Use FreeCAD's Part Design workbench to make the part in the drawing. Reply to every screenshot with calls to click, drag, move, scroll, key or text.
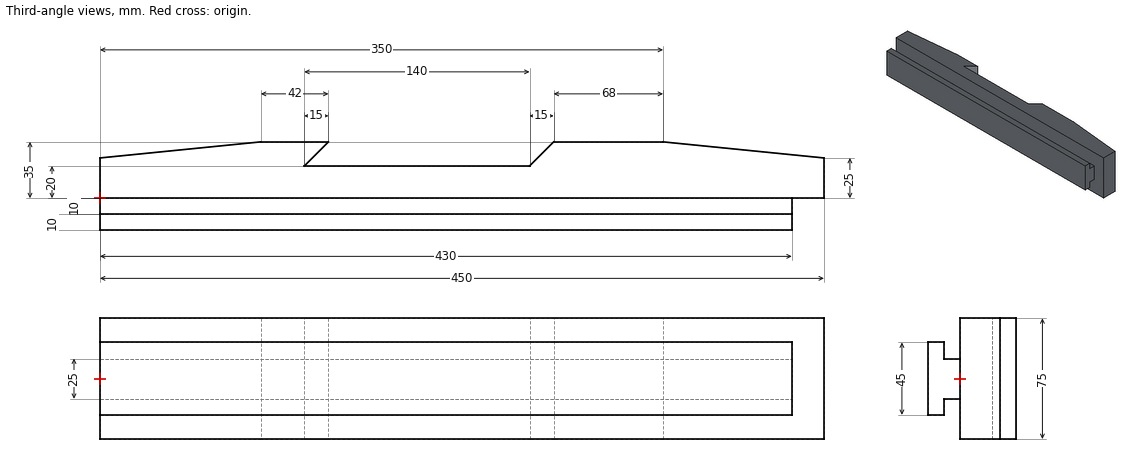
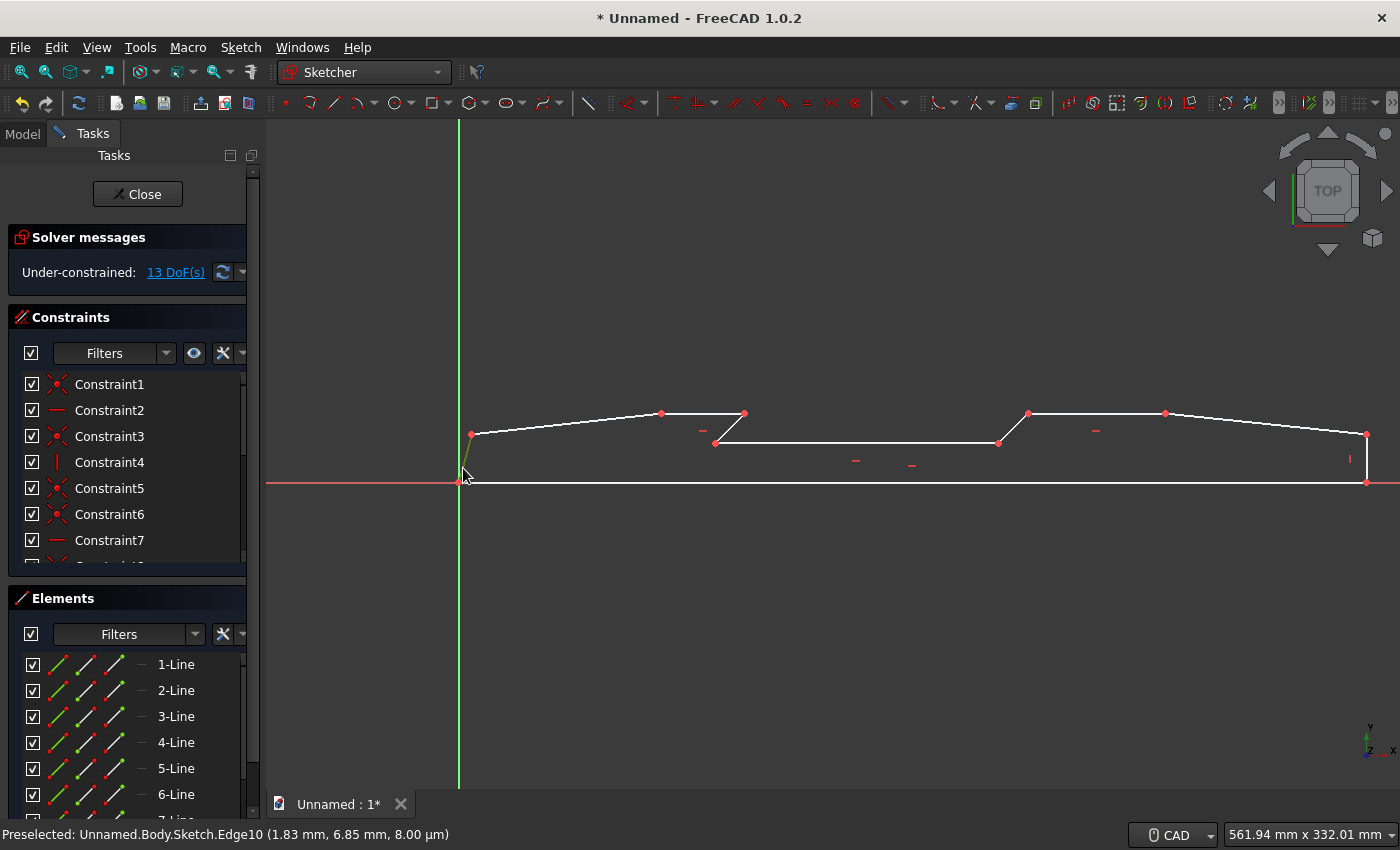
click(716, 104)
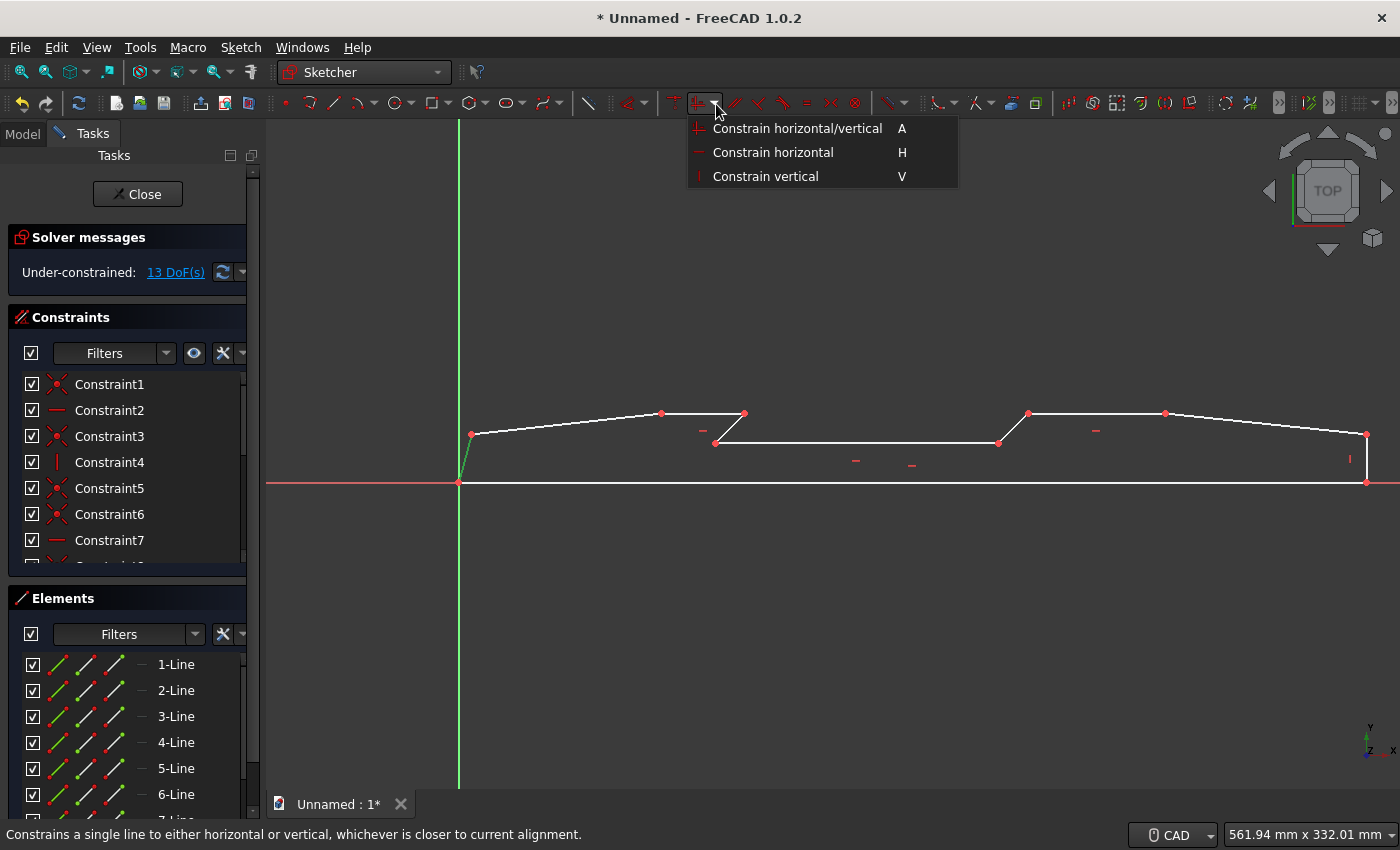
click(823, 176)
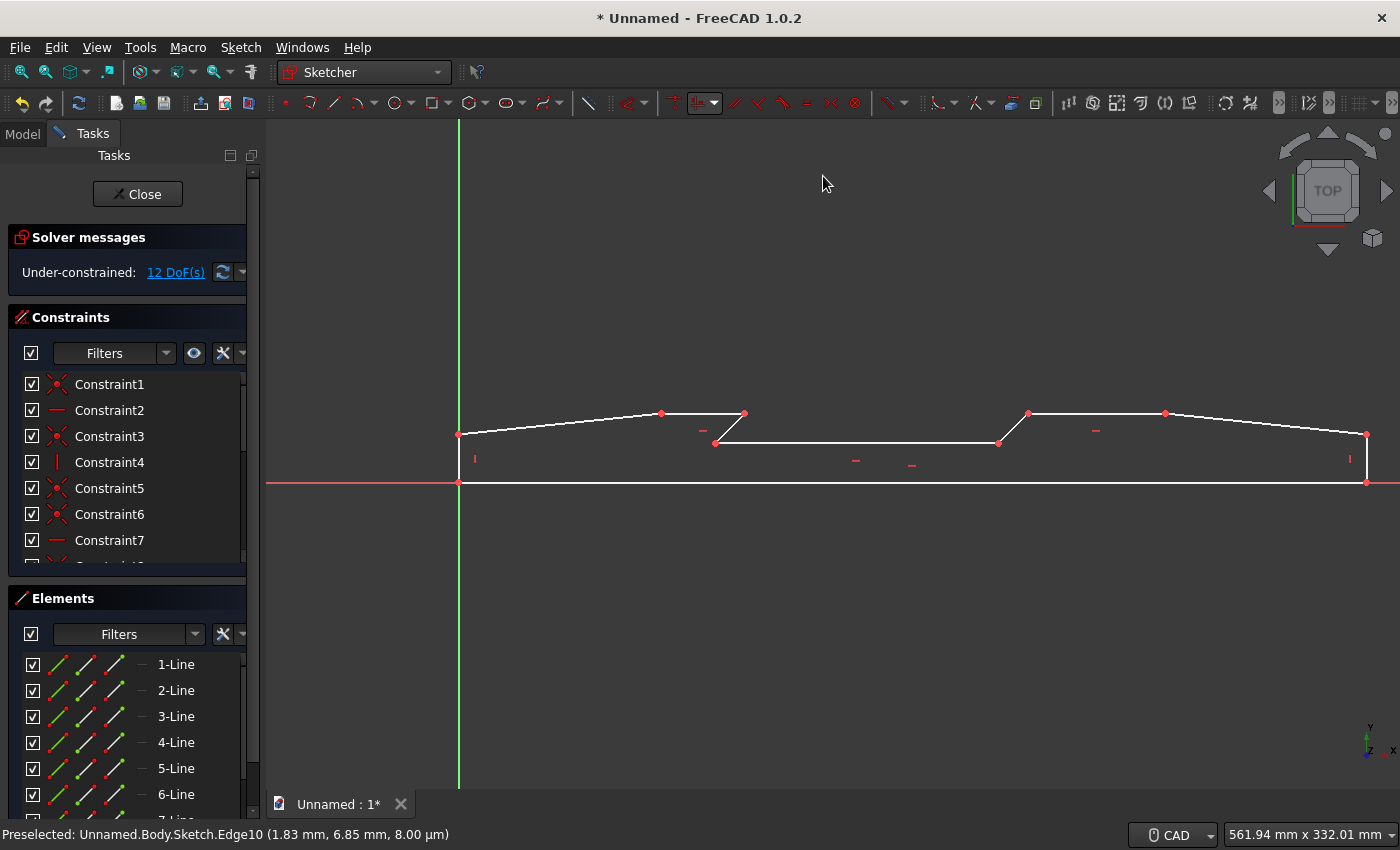
scroll(463, 467, down, 2)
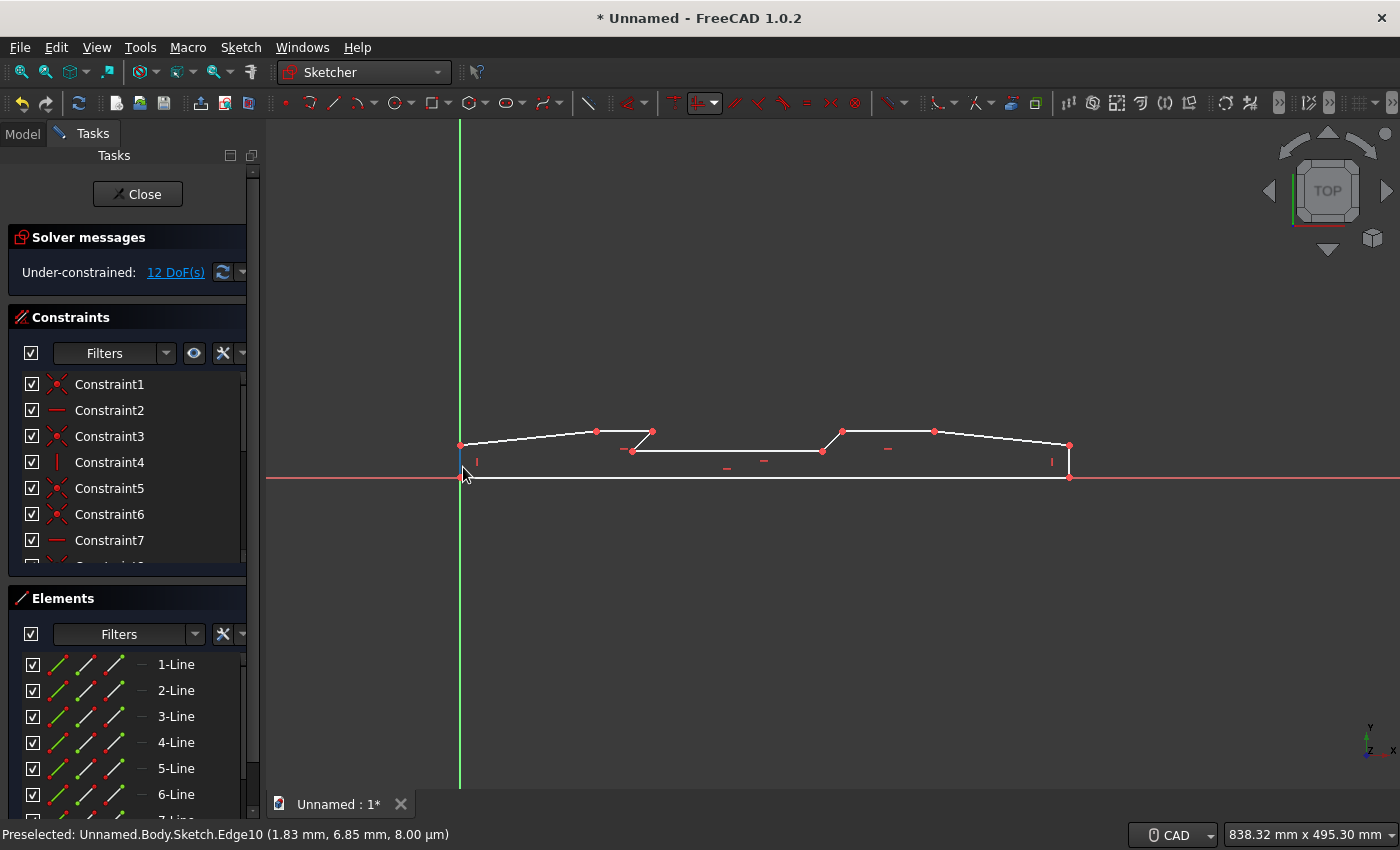
scroll(1069, 468, up, 2)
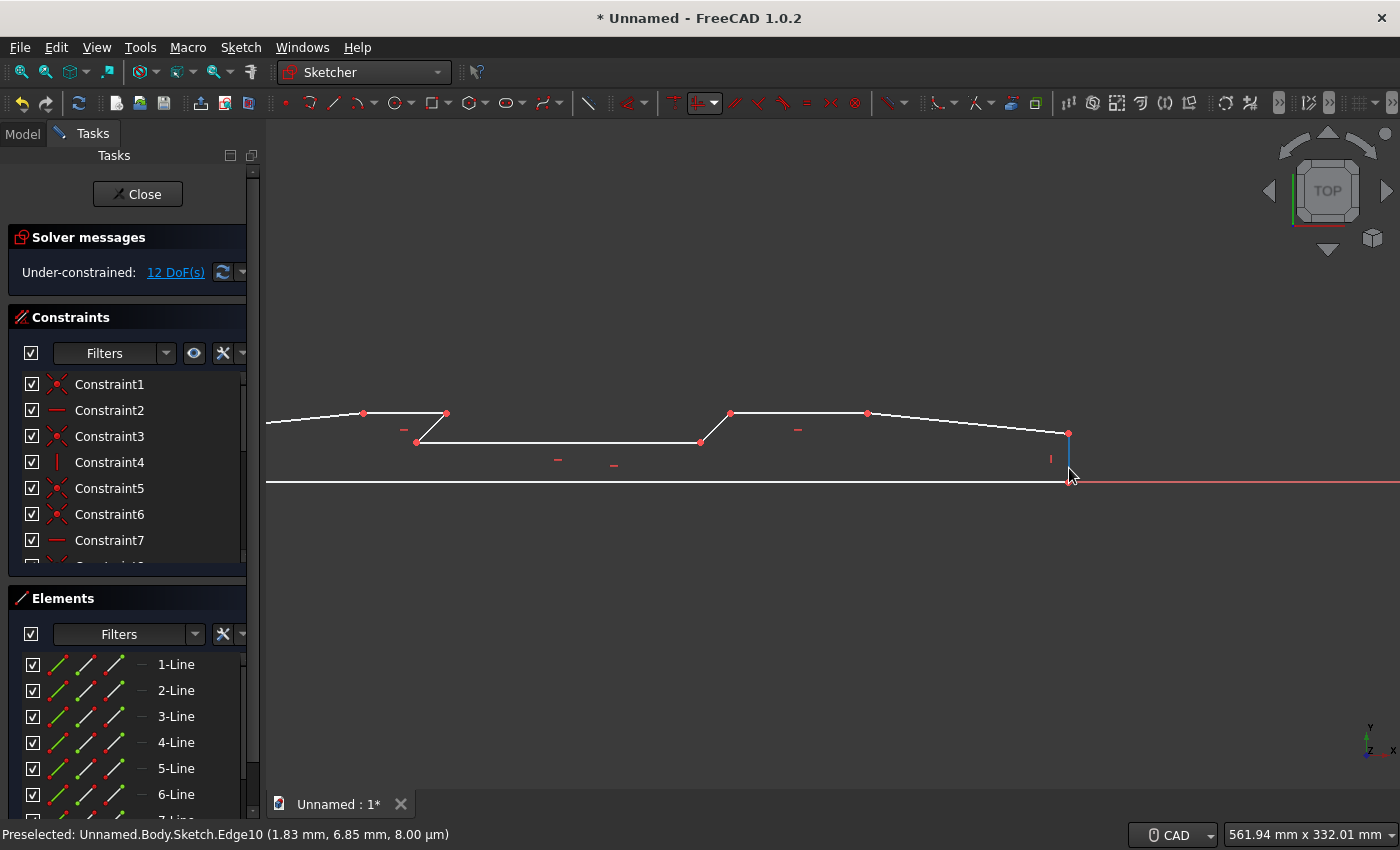
click(1069, 468)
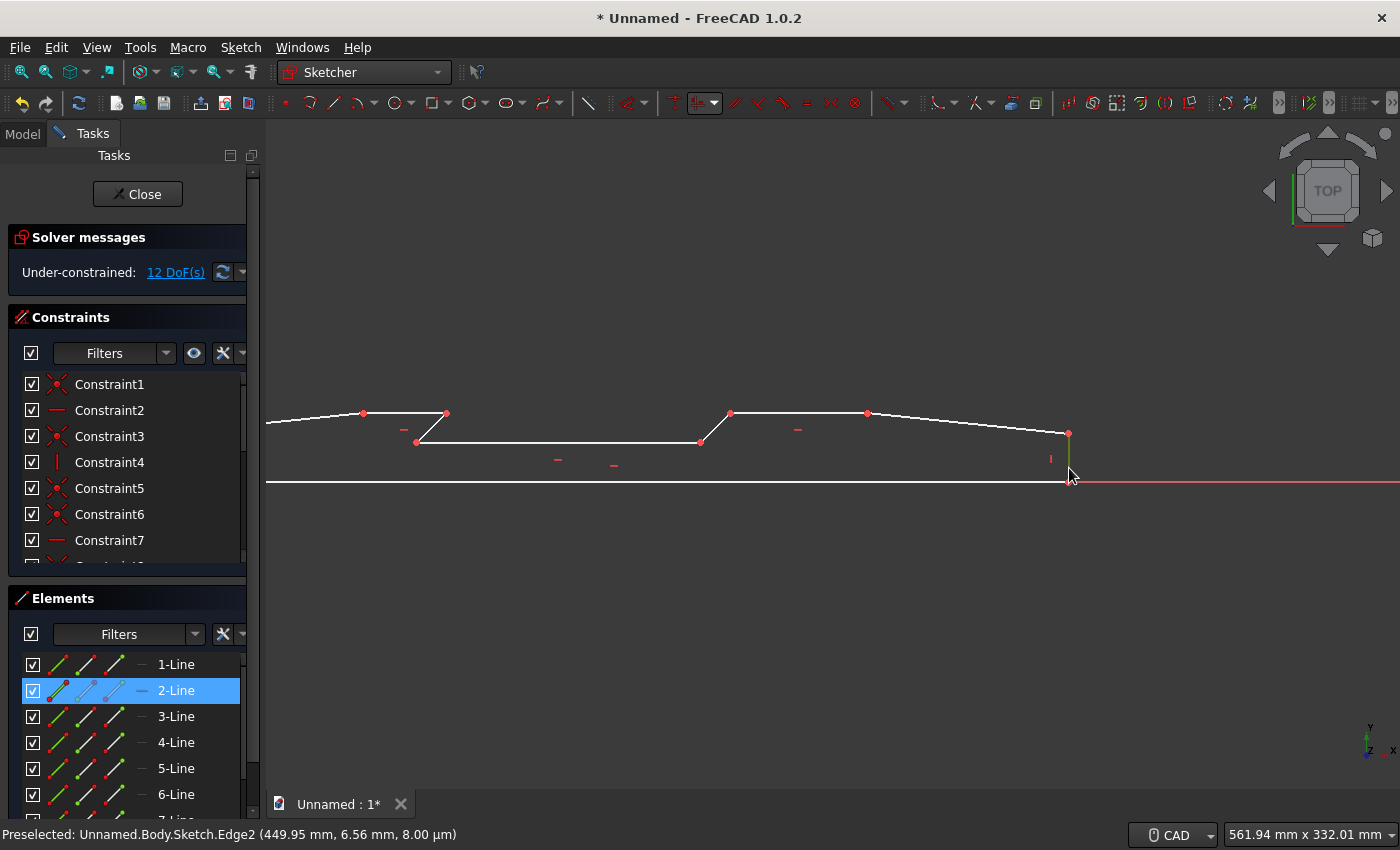
key(i)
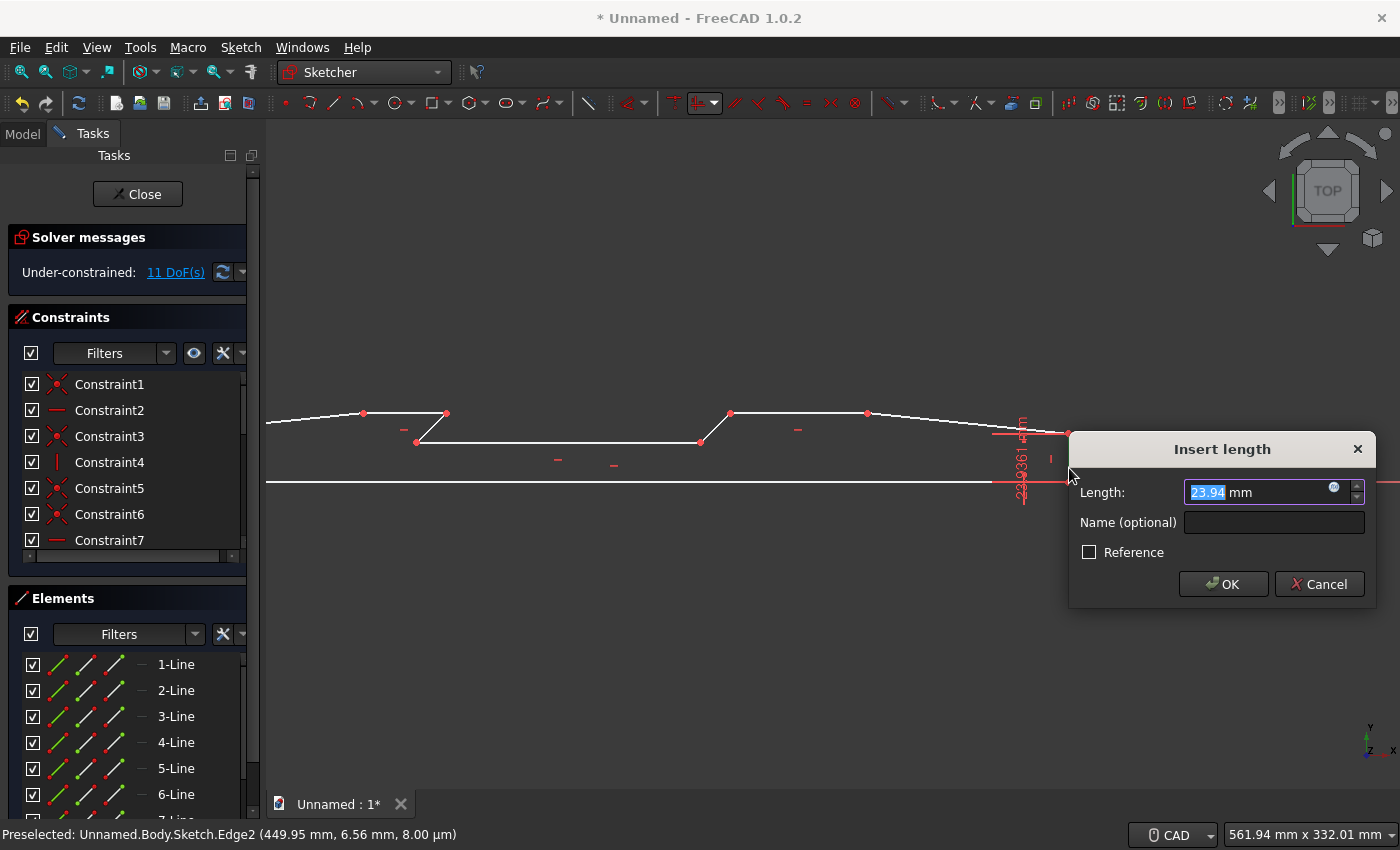
text(25)
key(Return)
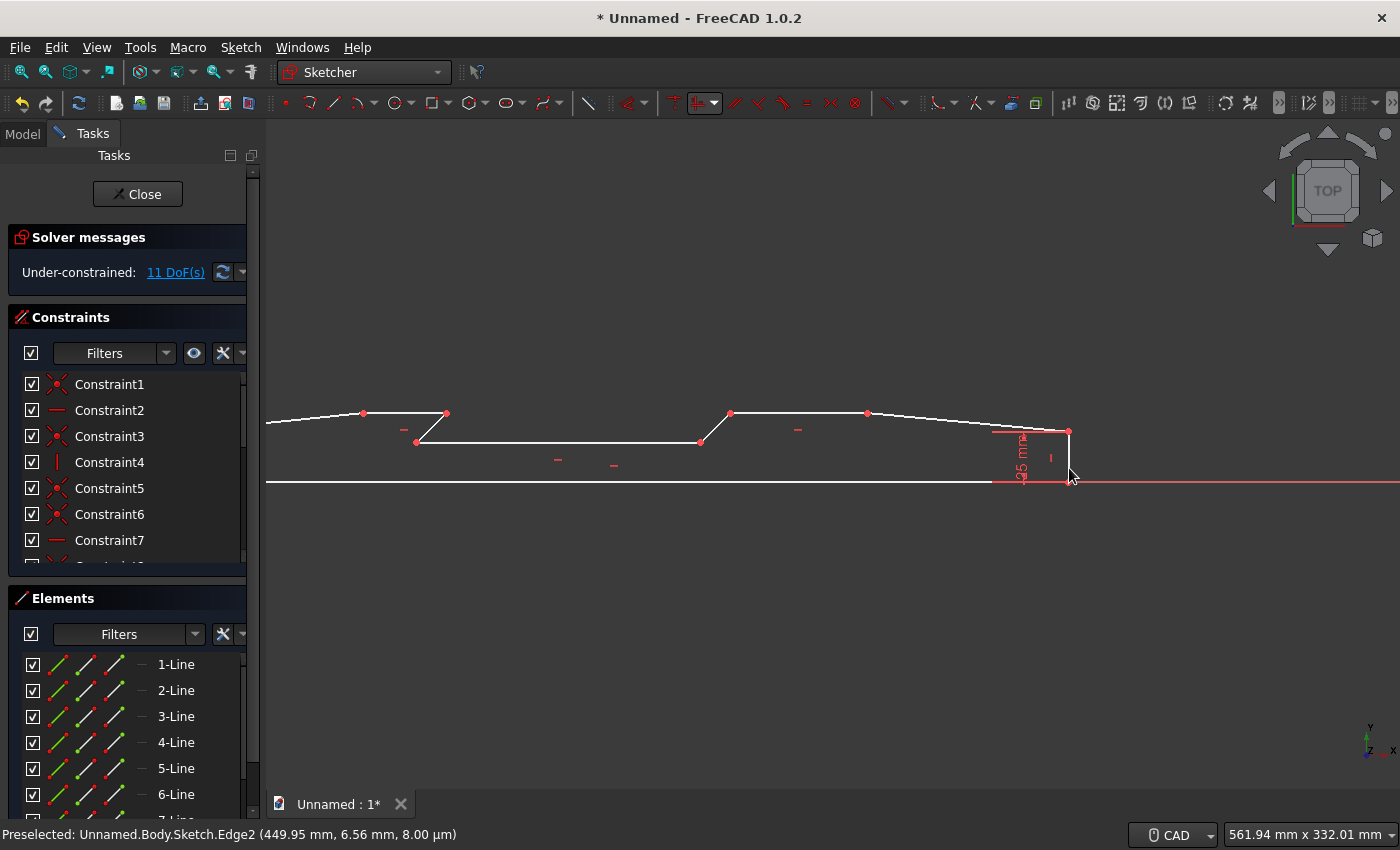
click(826, 413)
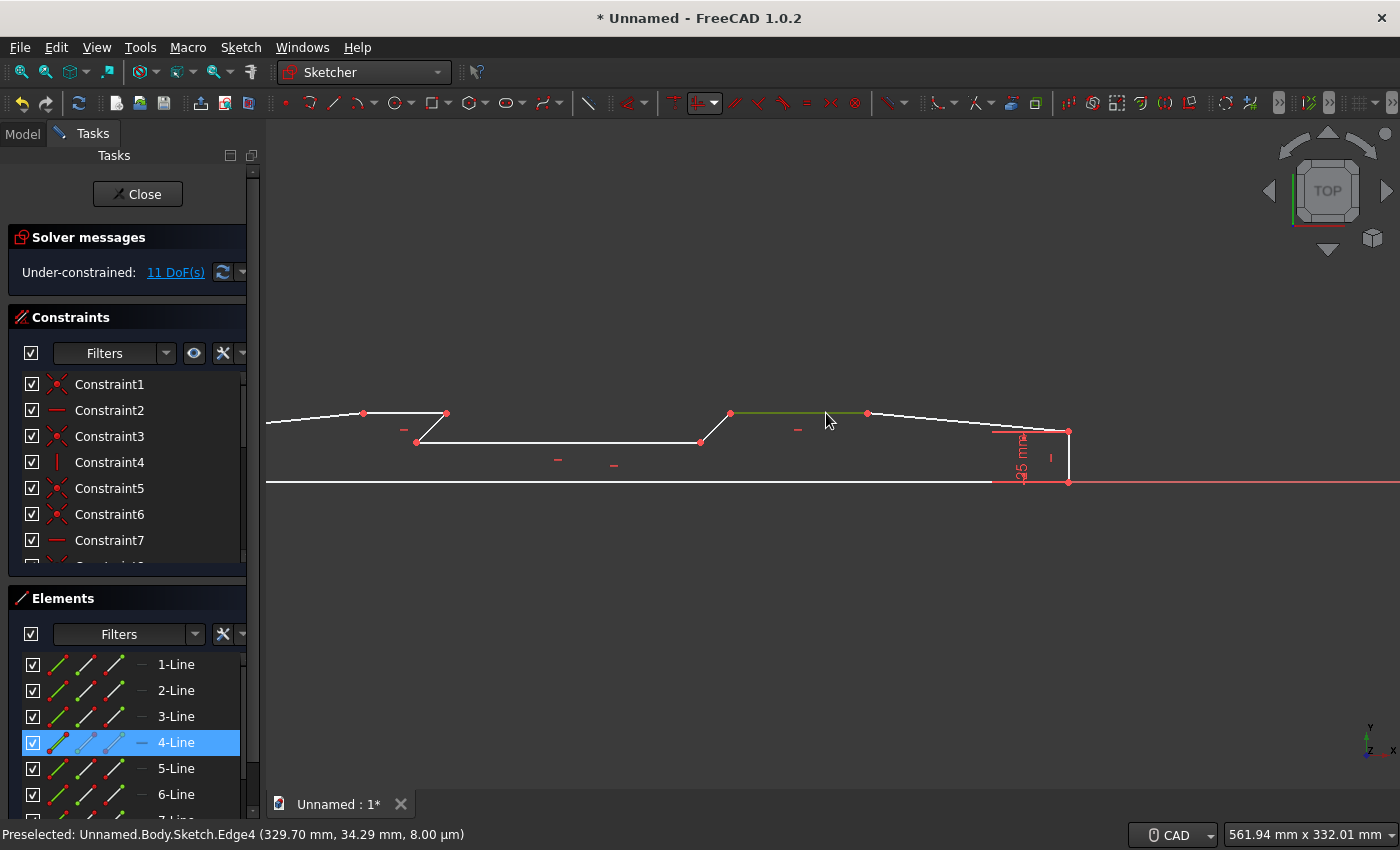
click(646, 104)